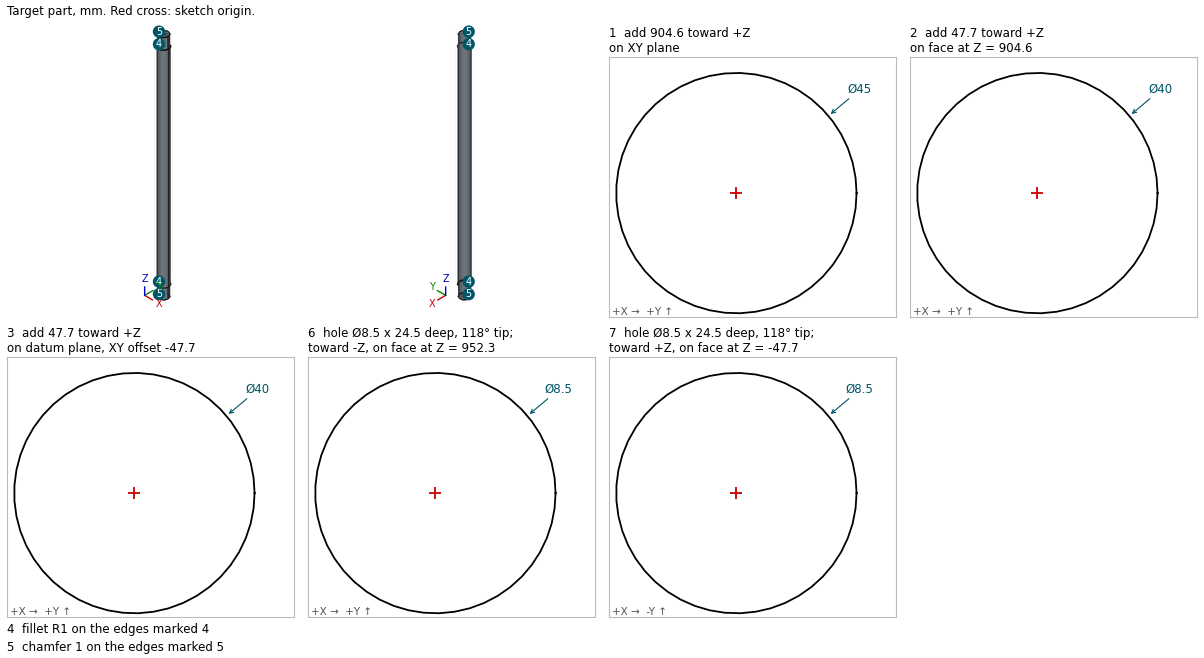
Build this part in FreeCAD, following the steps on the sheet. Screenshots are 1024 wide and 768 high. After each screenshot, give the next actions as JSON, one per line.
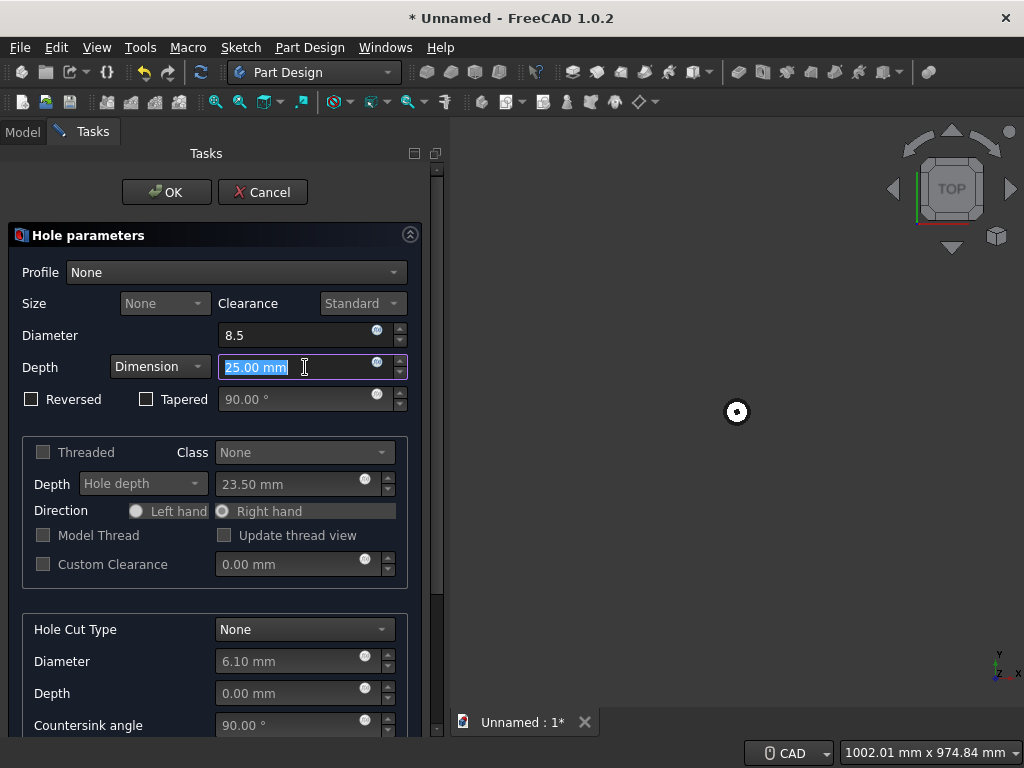
{"action": "type", "text": "24.5"}
{"action": "key", "text": "Tab"}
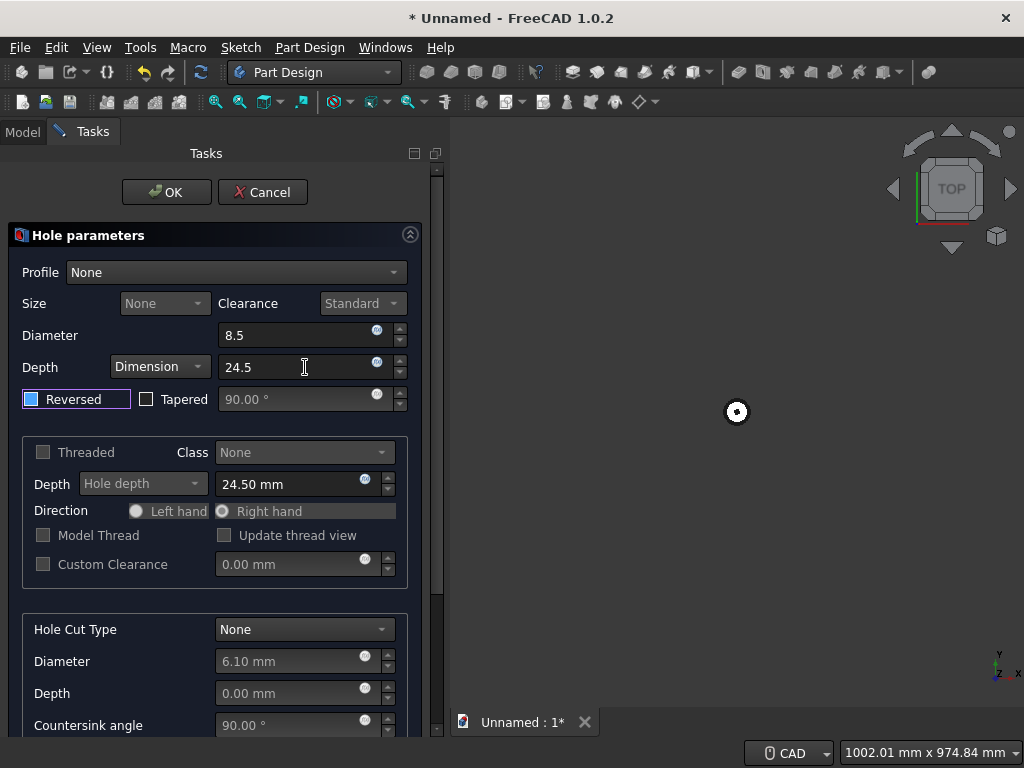
{"action": "left_click", "coordinate": [167, 192]}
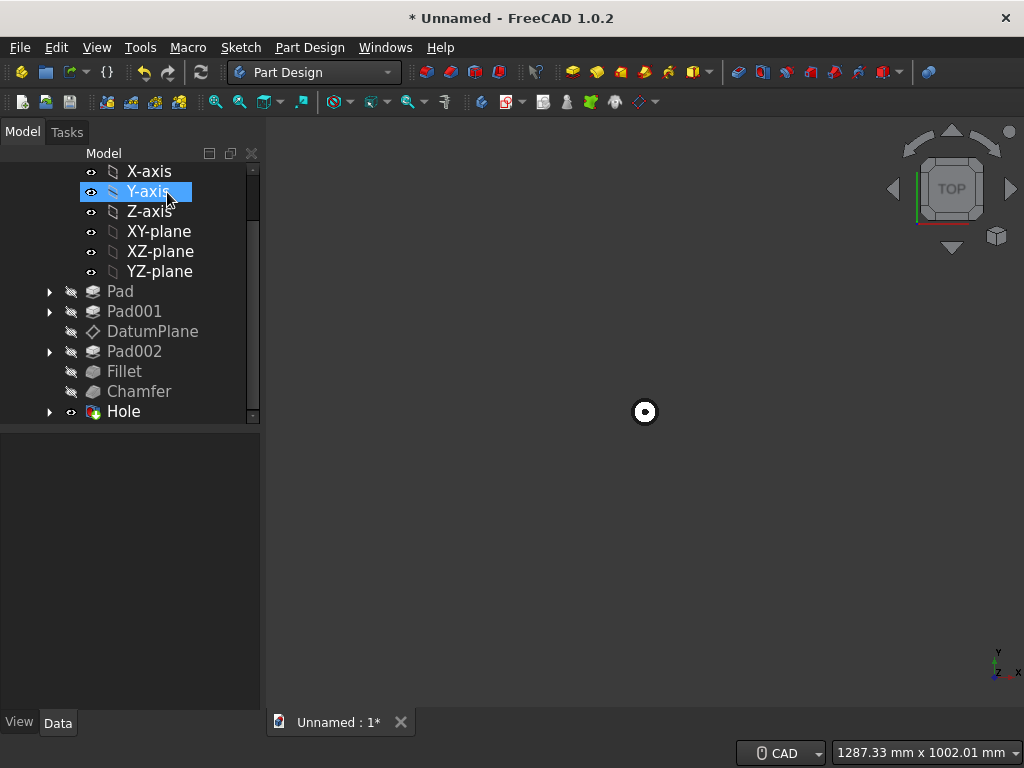
{"action": "key", "text": "v f"}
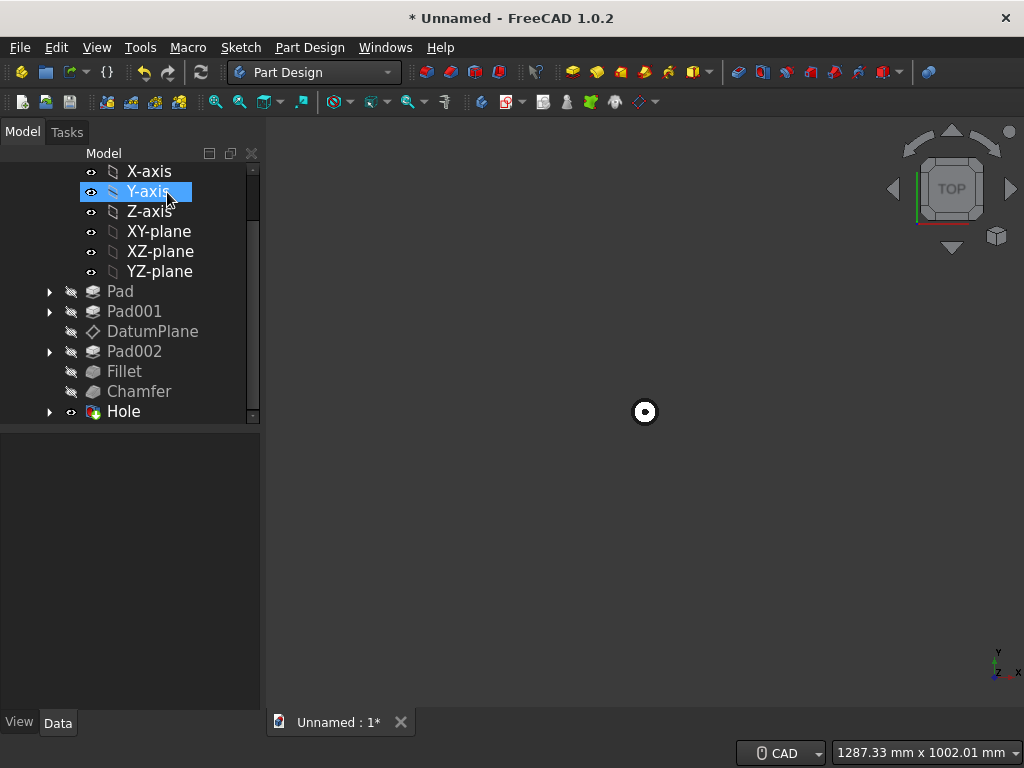
{"action": "key", "text": "5"}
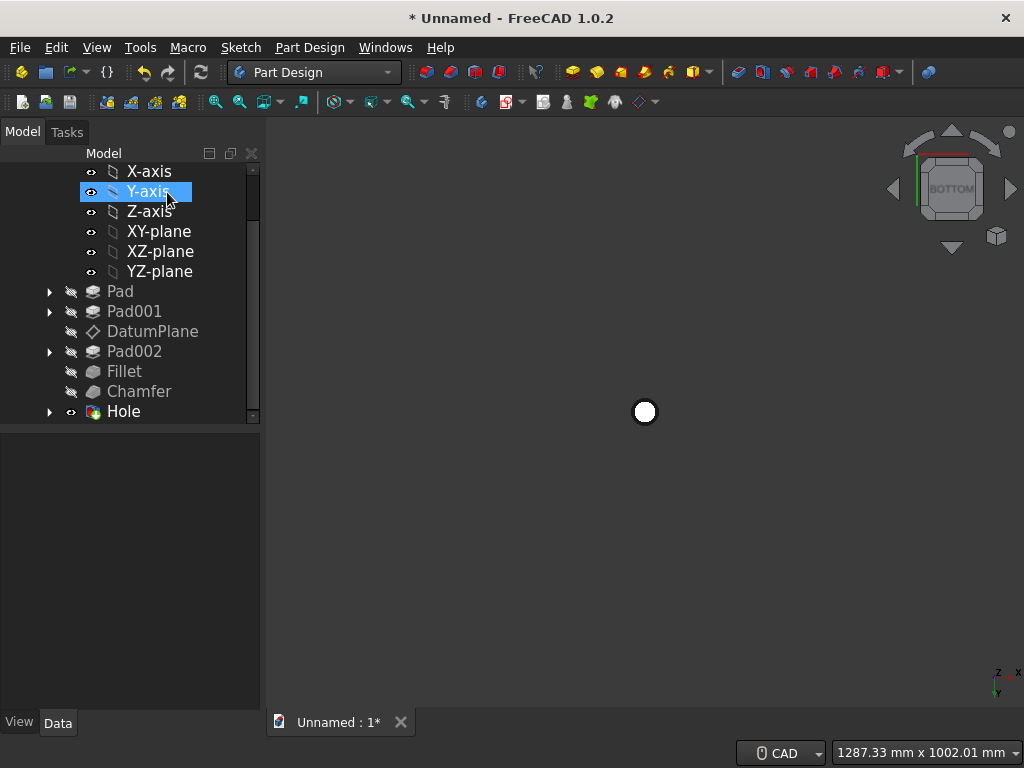
{"action": "key", "text": "v f"}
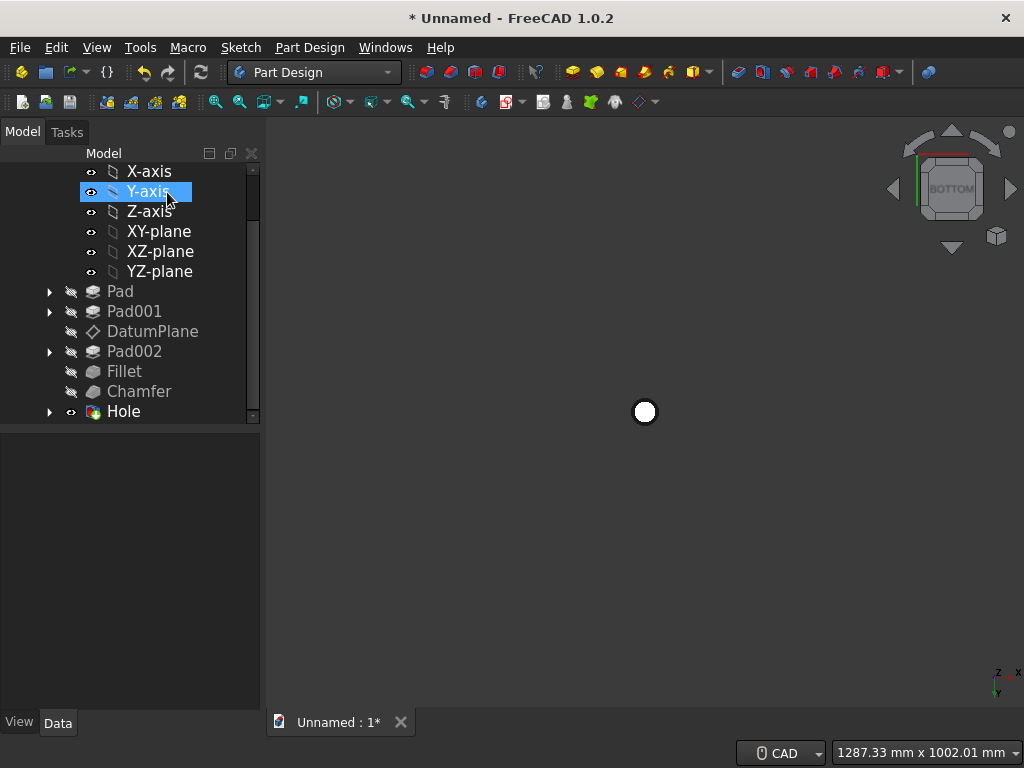
{"action": "left_click", "coordinate": [645, 411]}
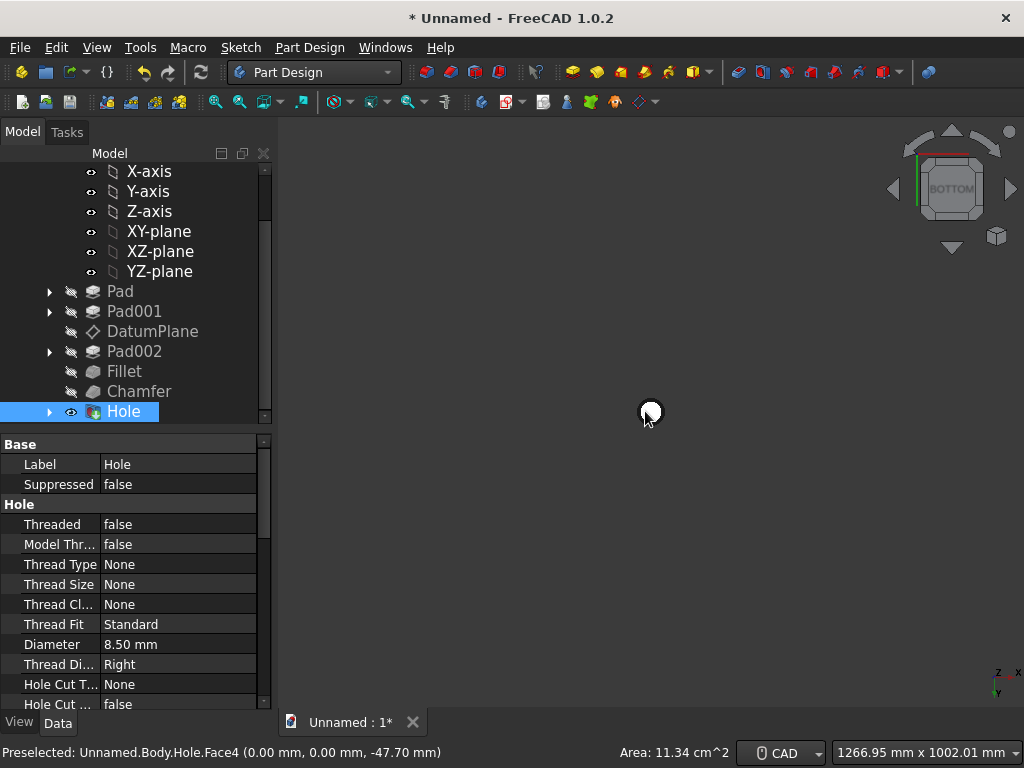
{"action": "left_click", "coordinate": [506, 102]}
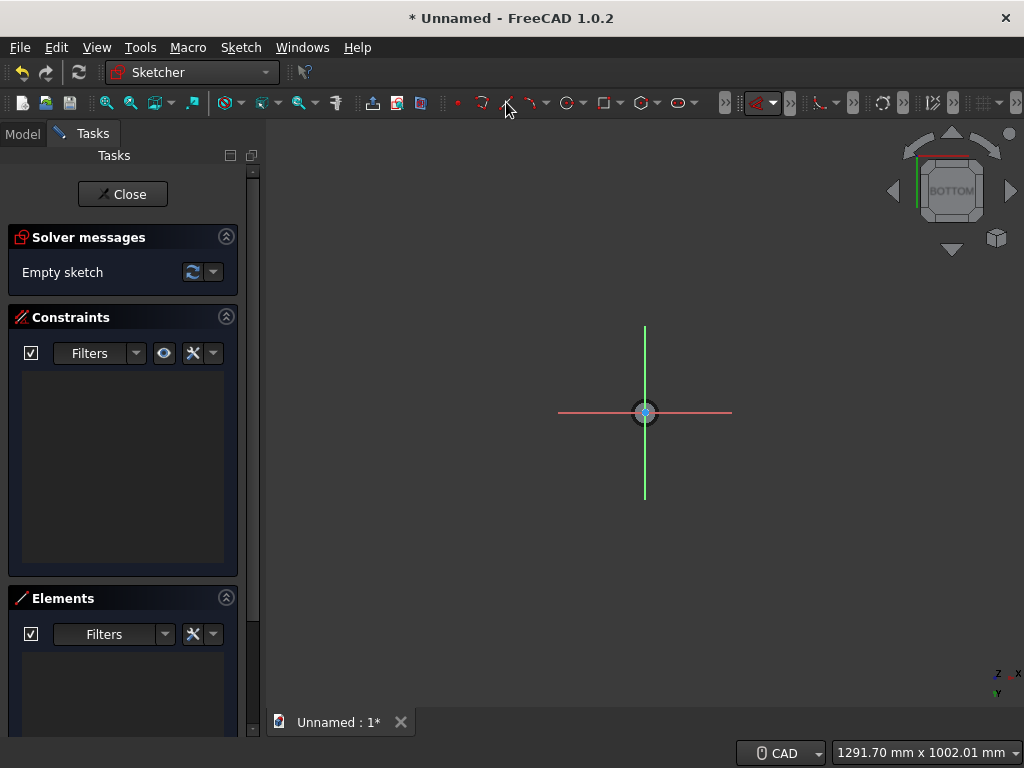
{"action": "scroll", "coordinate": [649, 413], "scroll_direction": "up", "scroll_amount": 15}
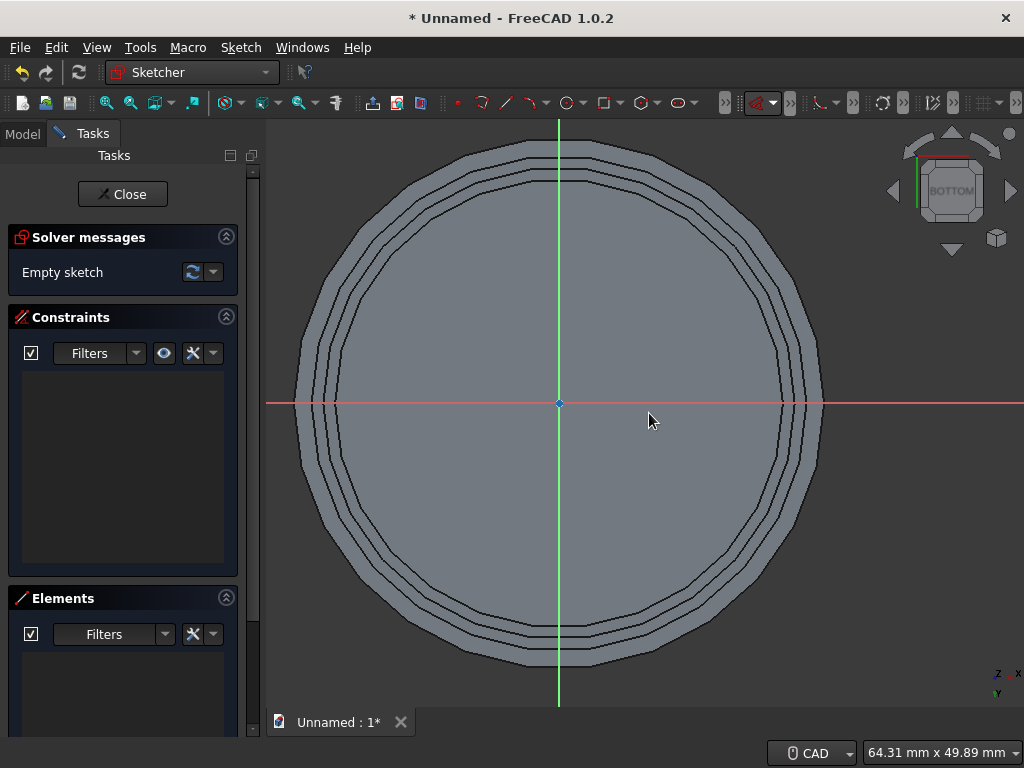
{"action": "scroll", "coordinate": [553, 400], "scroll_direction": "up", "scroll_amount": 7}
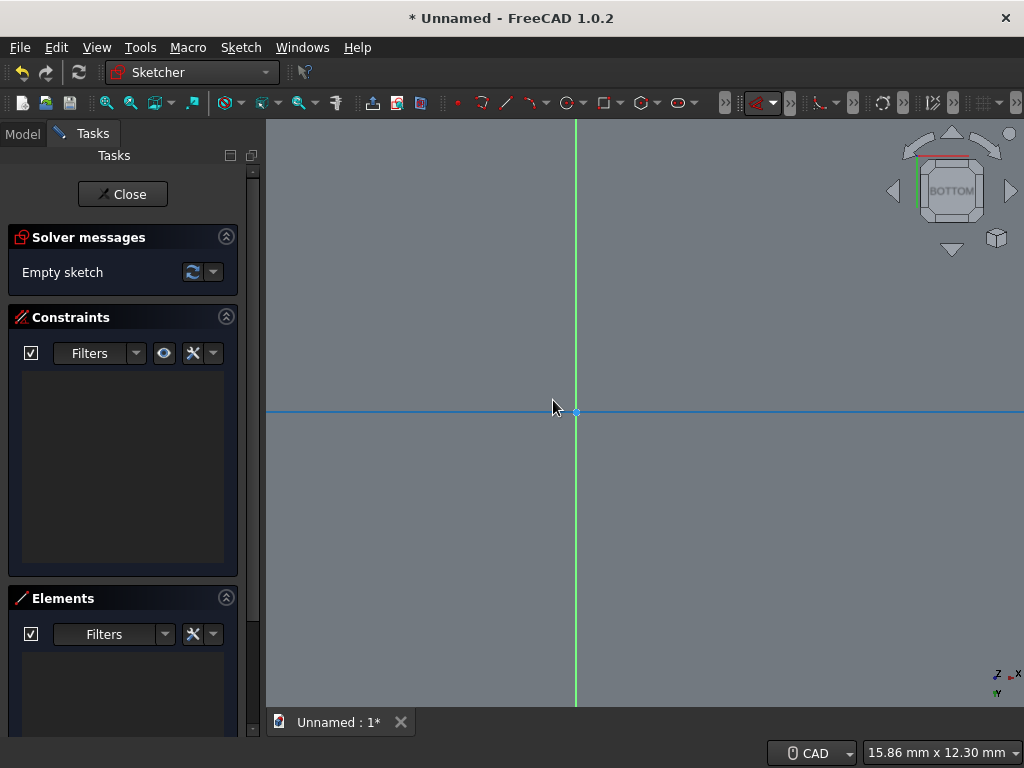
{"action": "key", "text": "g c"}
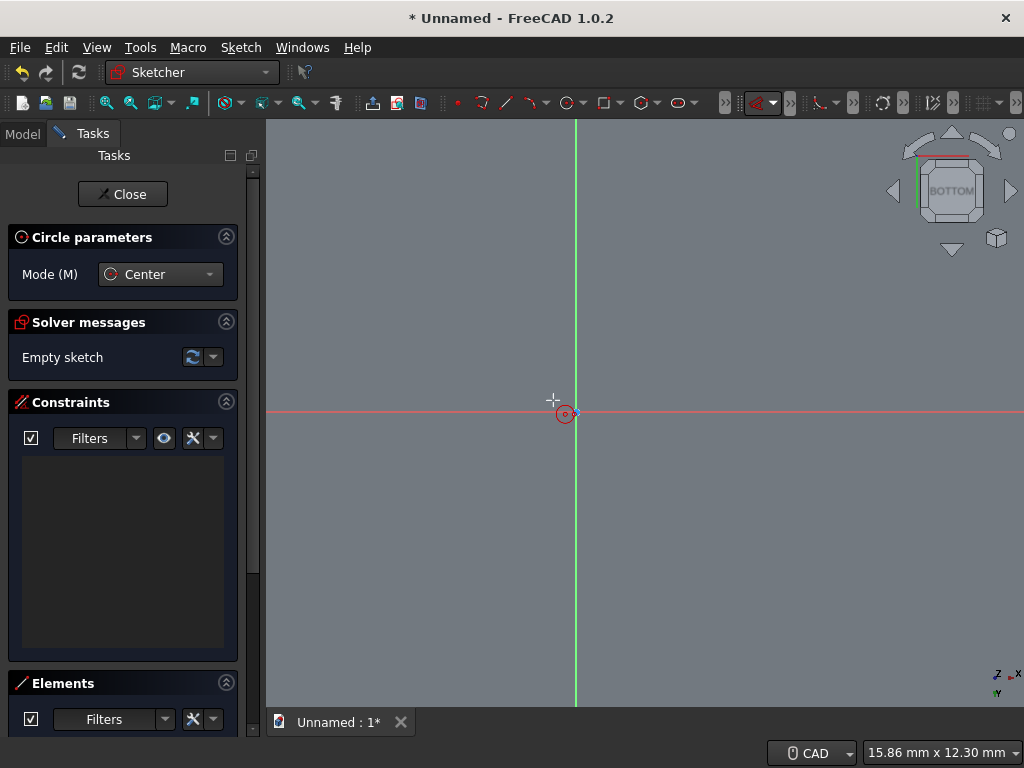
{"action": "left_click", "coordinate": [576, 412]}
{"action": "mouse_move", "coordinate": [720, 269]}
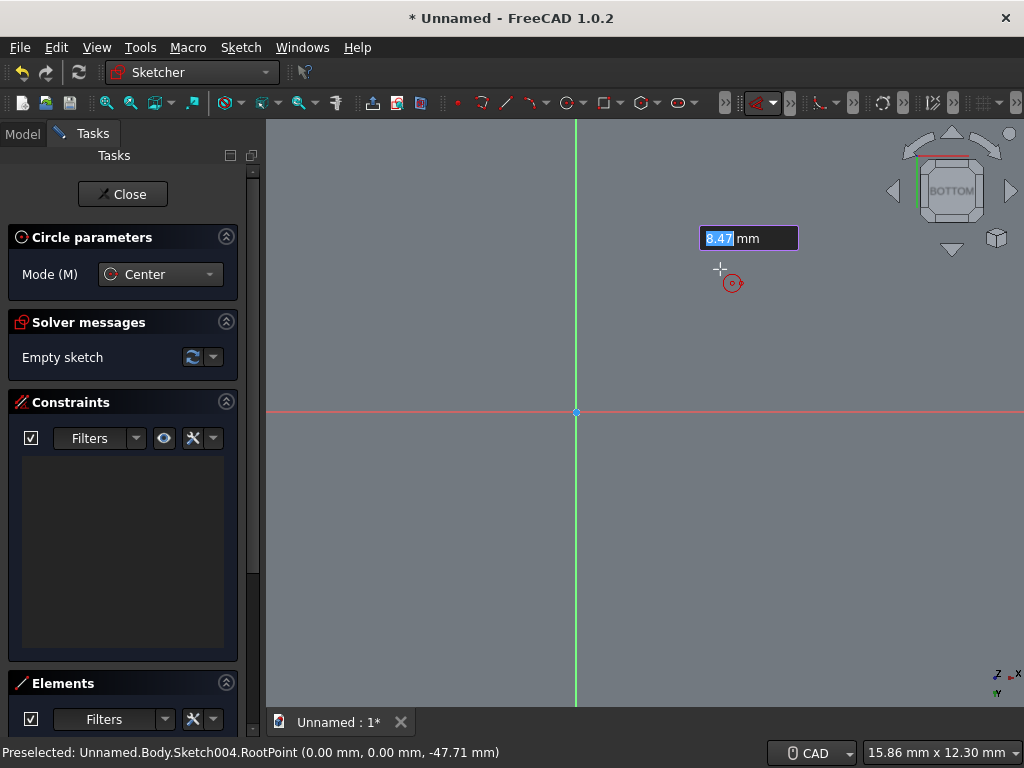
{"action": "type", "text": "8.5"}
{"action": "key", "text": "Return"}
{"action": "key", "text": "Escape"}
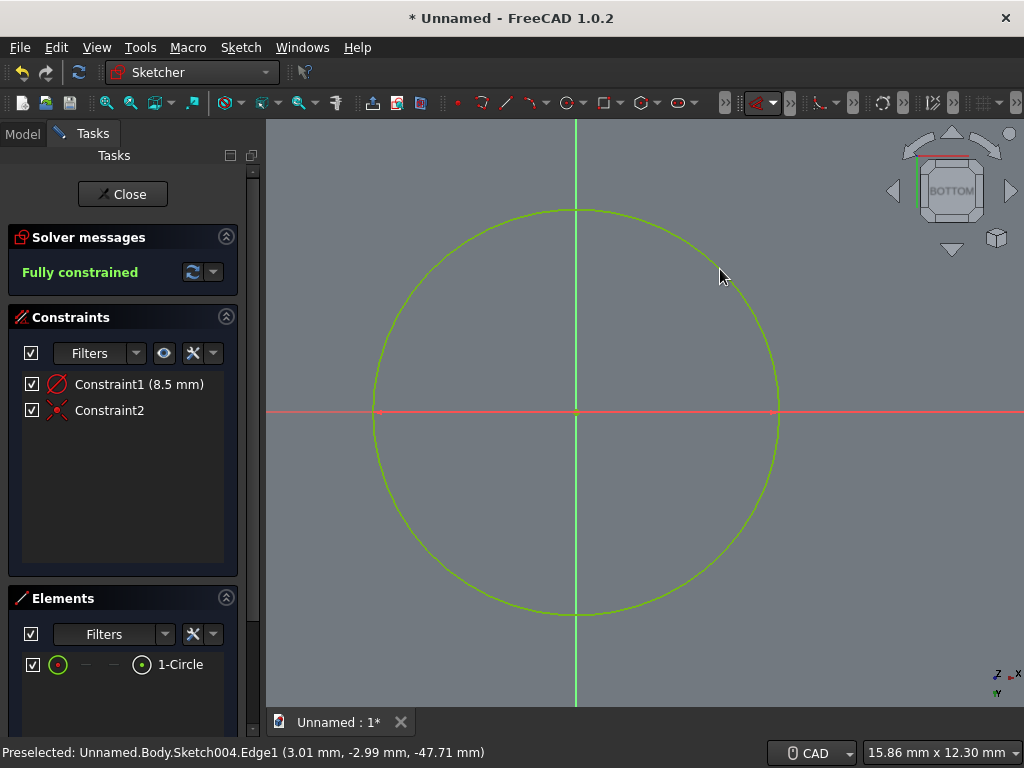
{"action": "left_click", "coordinate": [123, 194]}